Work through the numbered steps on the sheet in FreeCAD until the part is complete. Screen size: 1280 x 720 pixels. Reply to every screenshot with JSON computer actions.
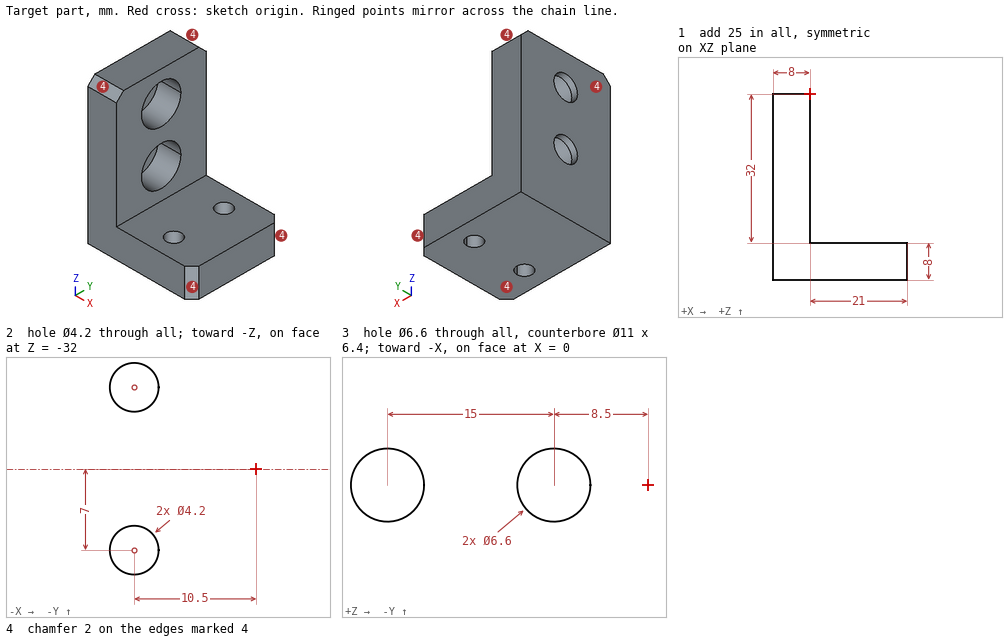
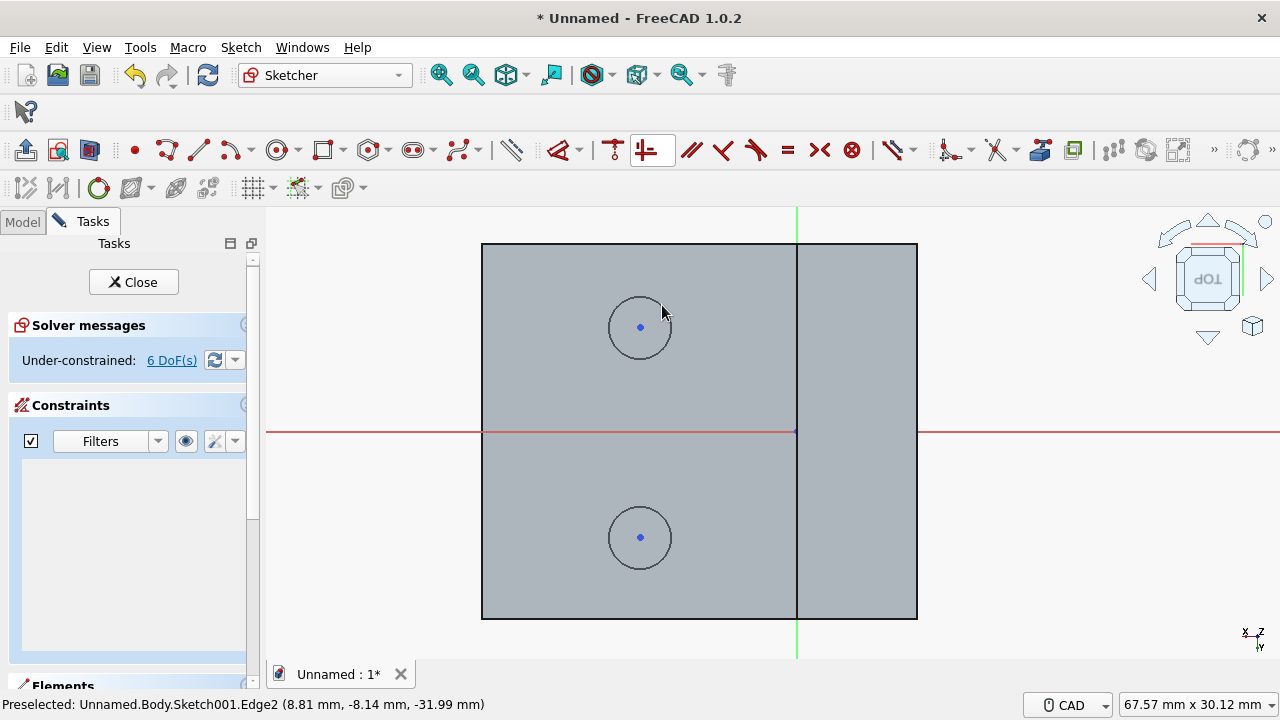
{"action": "left_click", "coordinate": [662, 516]}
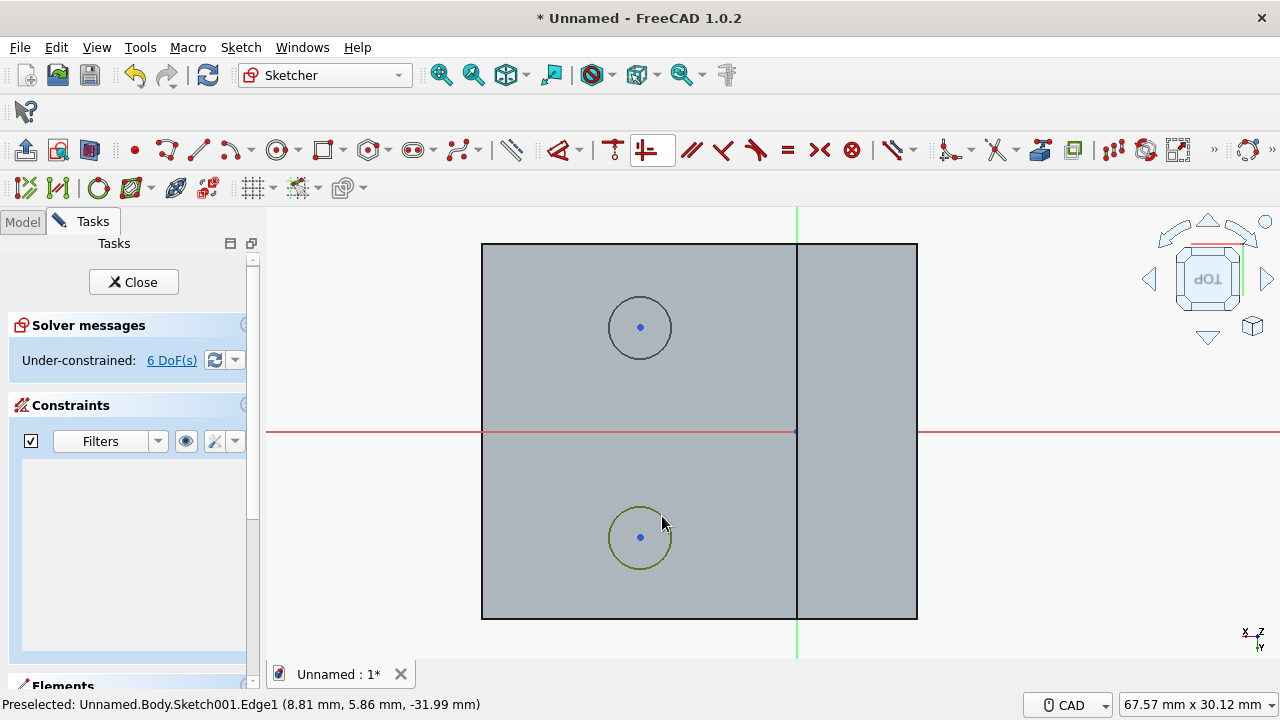
{"action": "left_click", "coordinate": [662, 306]}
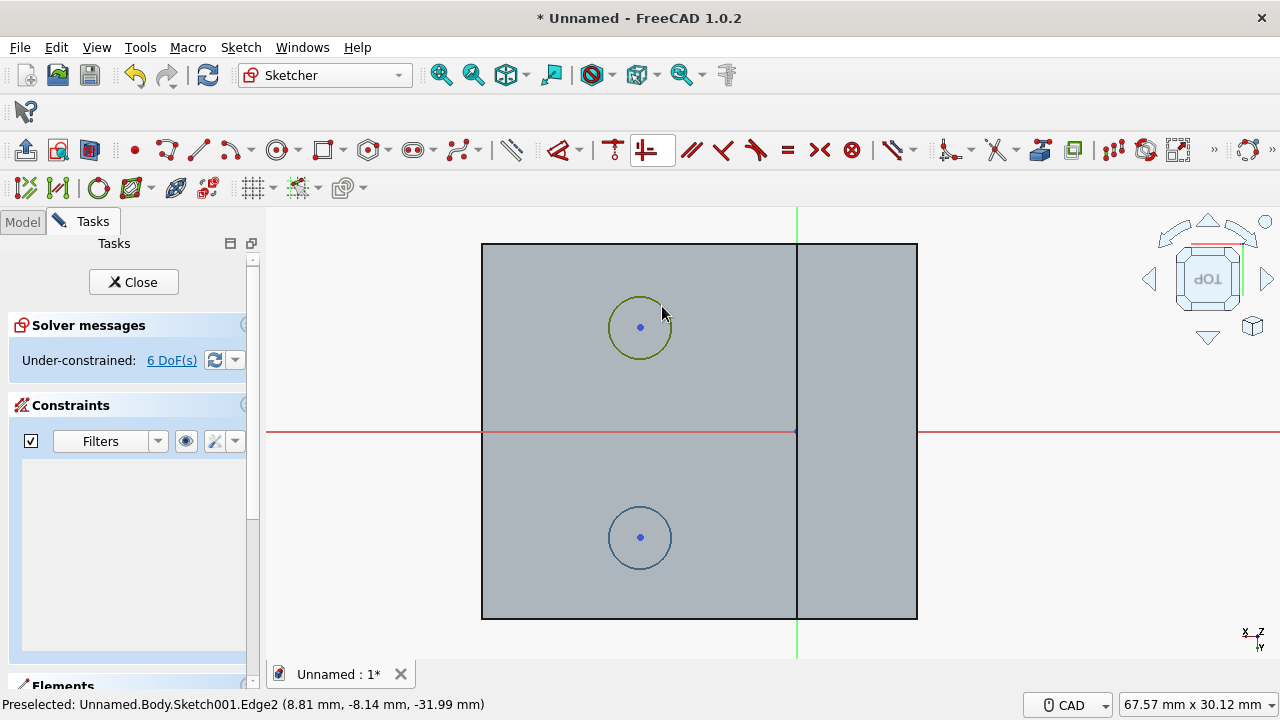
{"action": "left_click", "coordinate": [788, 150]}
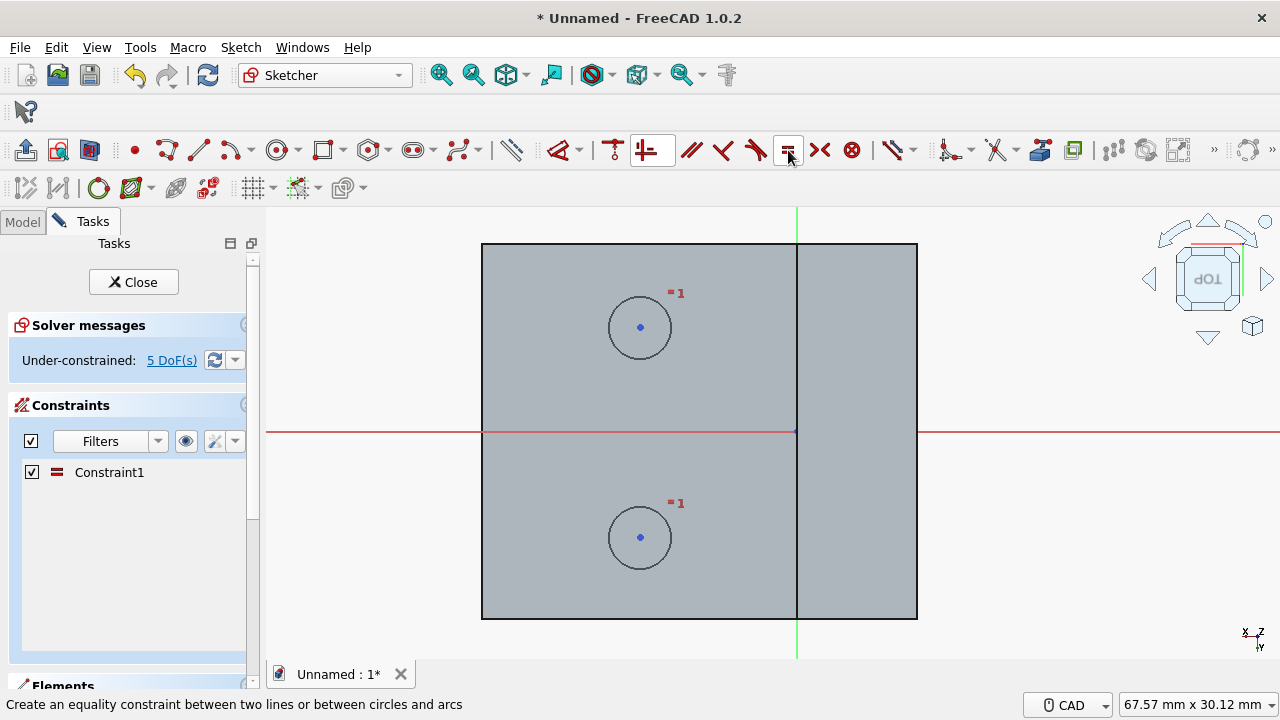
{"action": "left_click", "coordinate": [640, 538]}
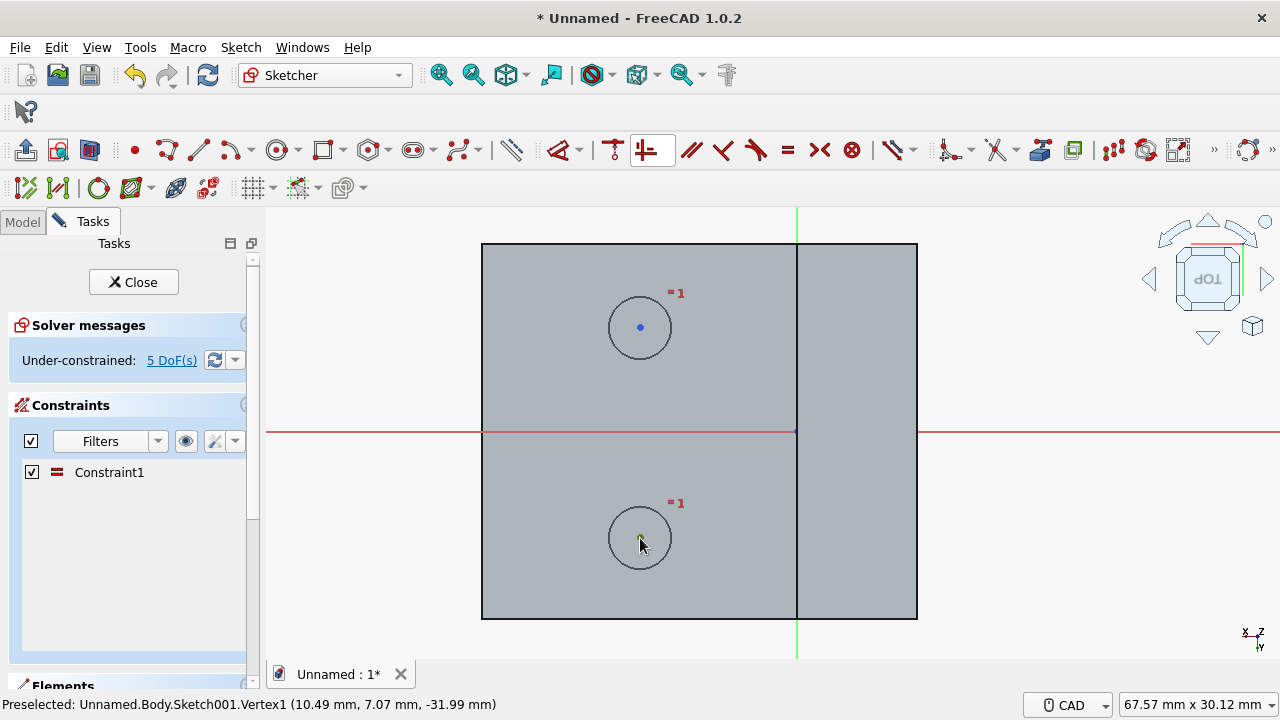
{"action": "left_click", "coordinate": [640, 328]}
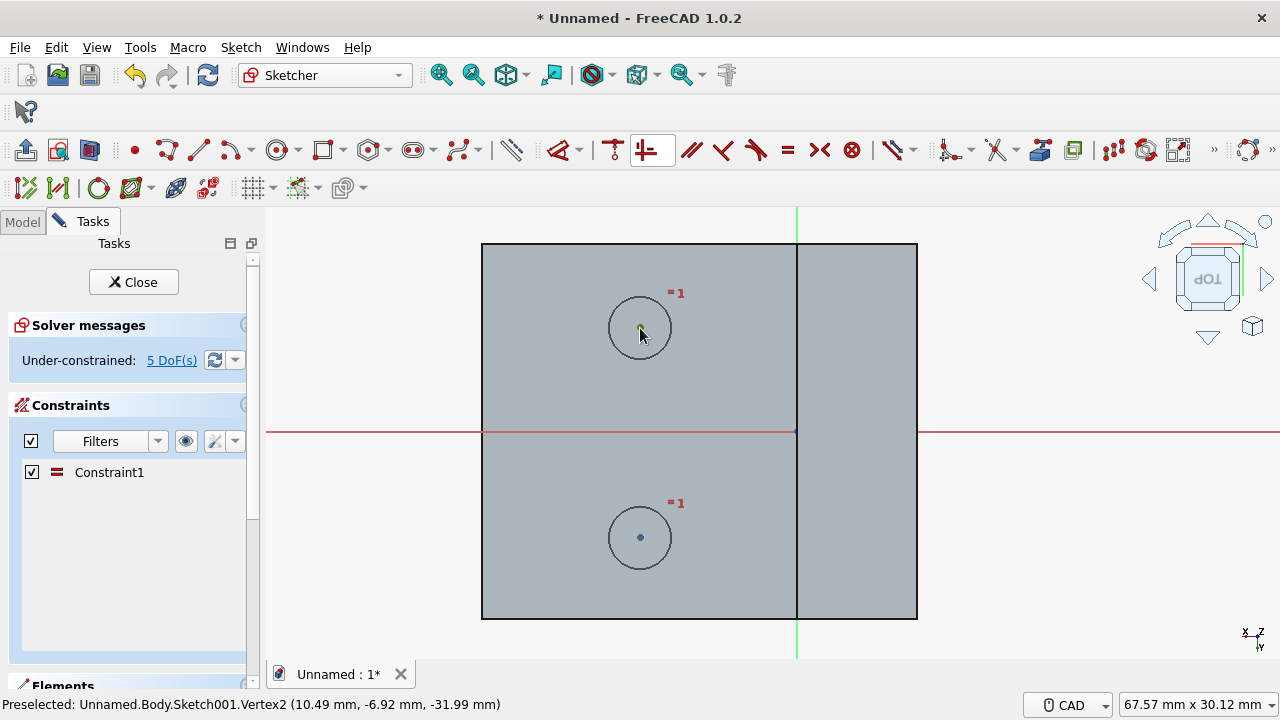
{"action": "left_click", "coordinate": [353, 432]}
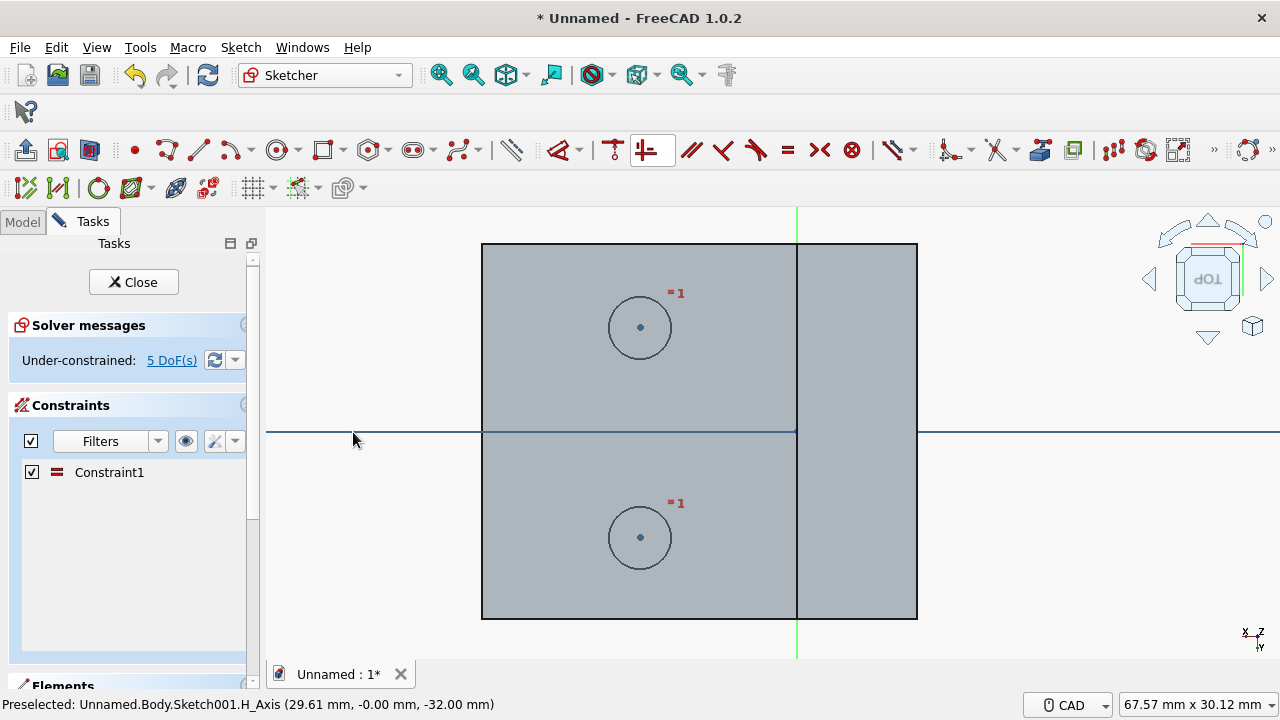
{"action": "left_click", "coordinate": [820, 150]}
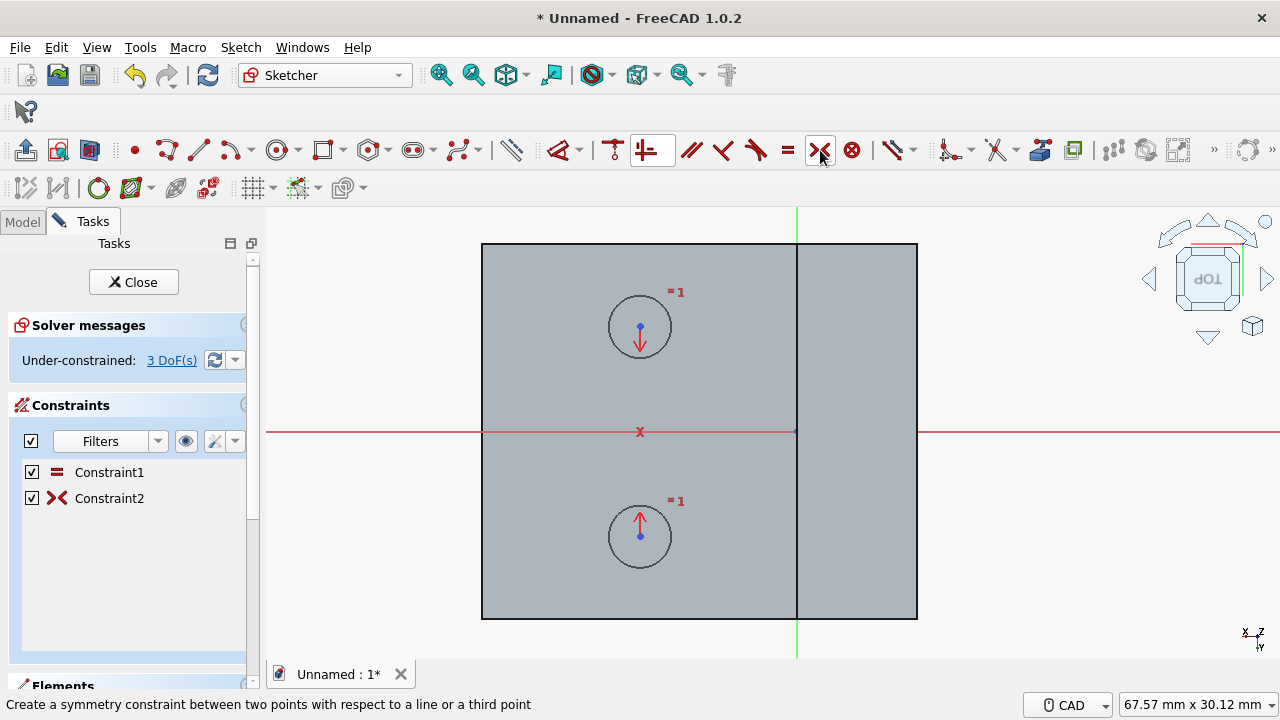
{"action": "left_click", "coordinate": [558, 150]}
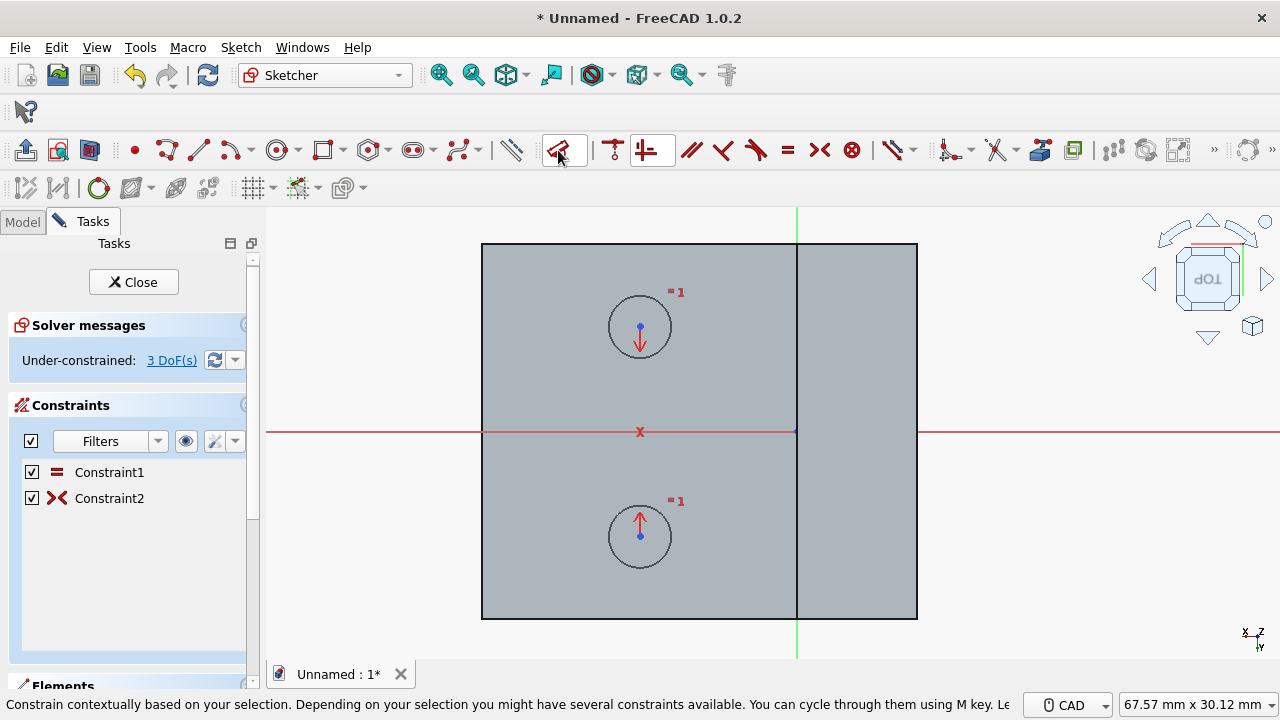
{"action": "left_click", "coordinate": [662, 515]}
{"action": "left_click", "coordinate": [685, 493]}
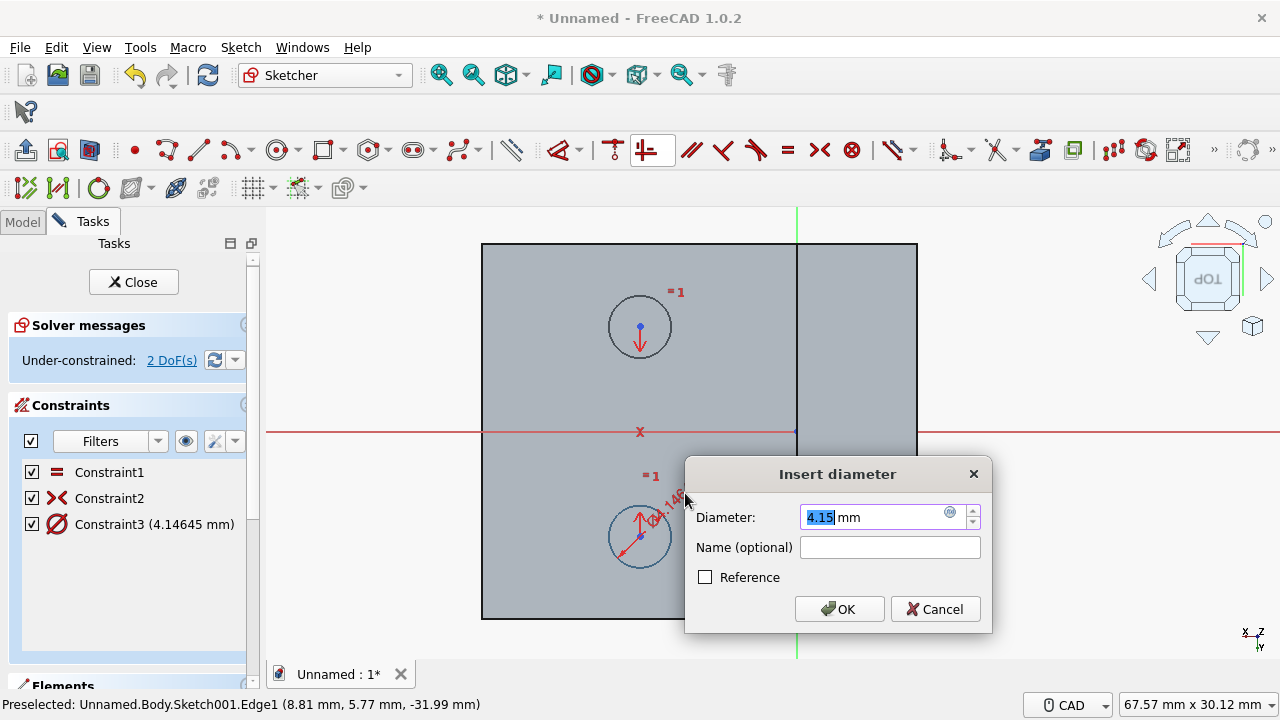
{"action": "type", "text": "4.2"}
{"action": "key", "text": "Return"}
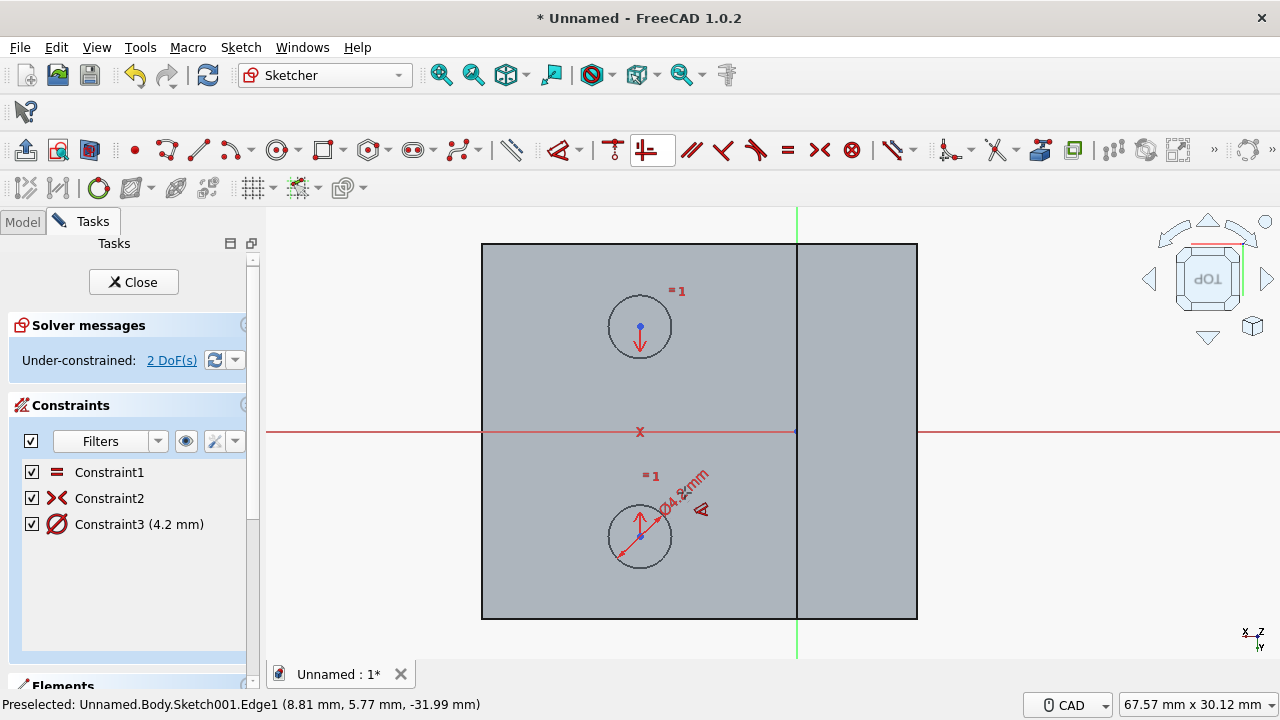
{"action": "left_click", "coordinate": [640, 537]}
{"action": "left_click", "coordinate": [831, 484]}